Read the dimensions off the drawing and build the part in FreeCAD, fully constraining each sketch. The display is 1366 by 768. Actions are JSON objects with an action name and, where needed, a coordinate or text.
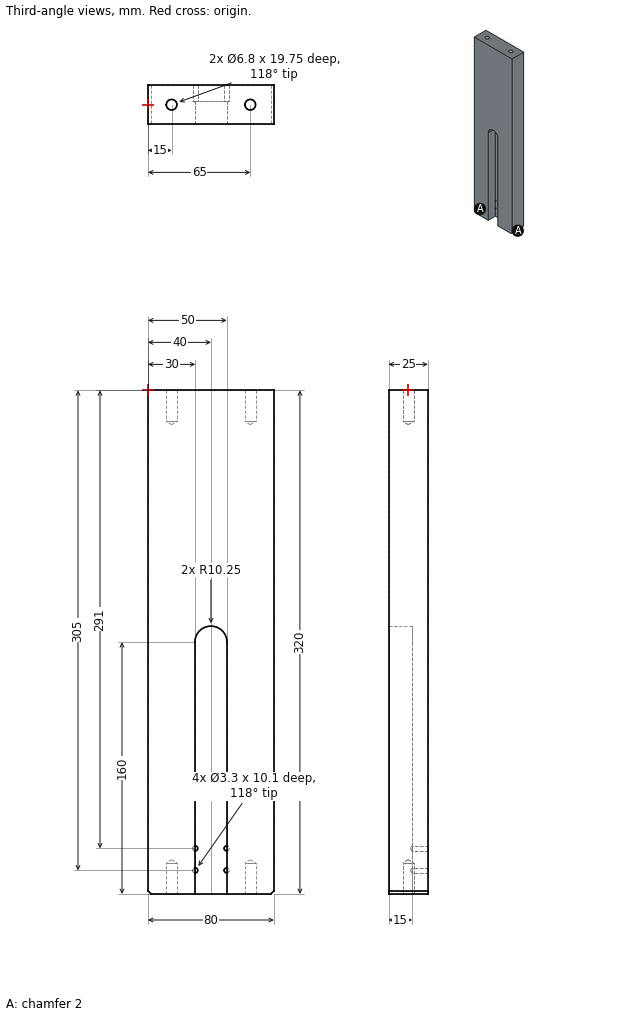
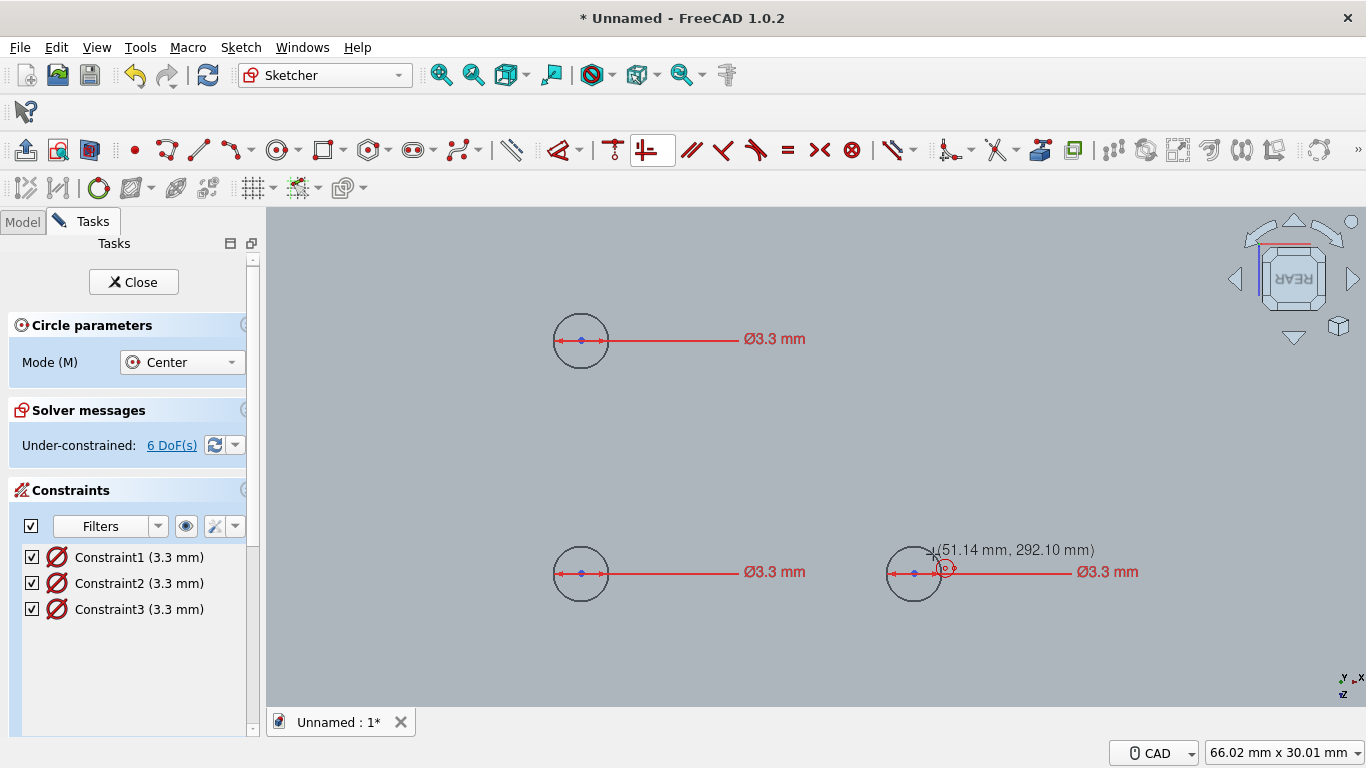
{"action": "left_click", "coordinate": [914, 340]}
{"action": "mouse_move", "coordinate": [933, 321]}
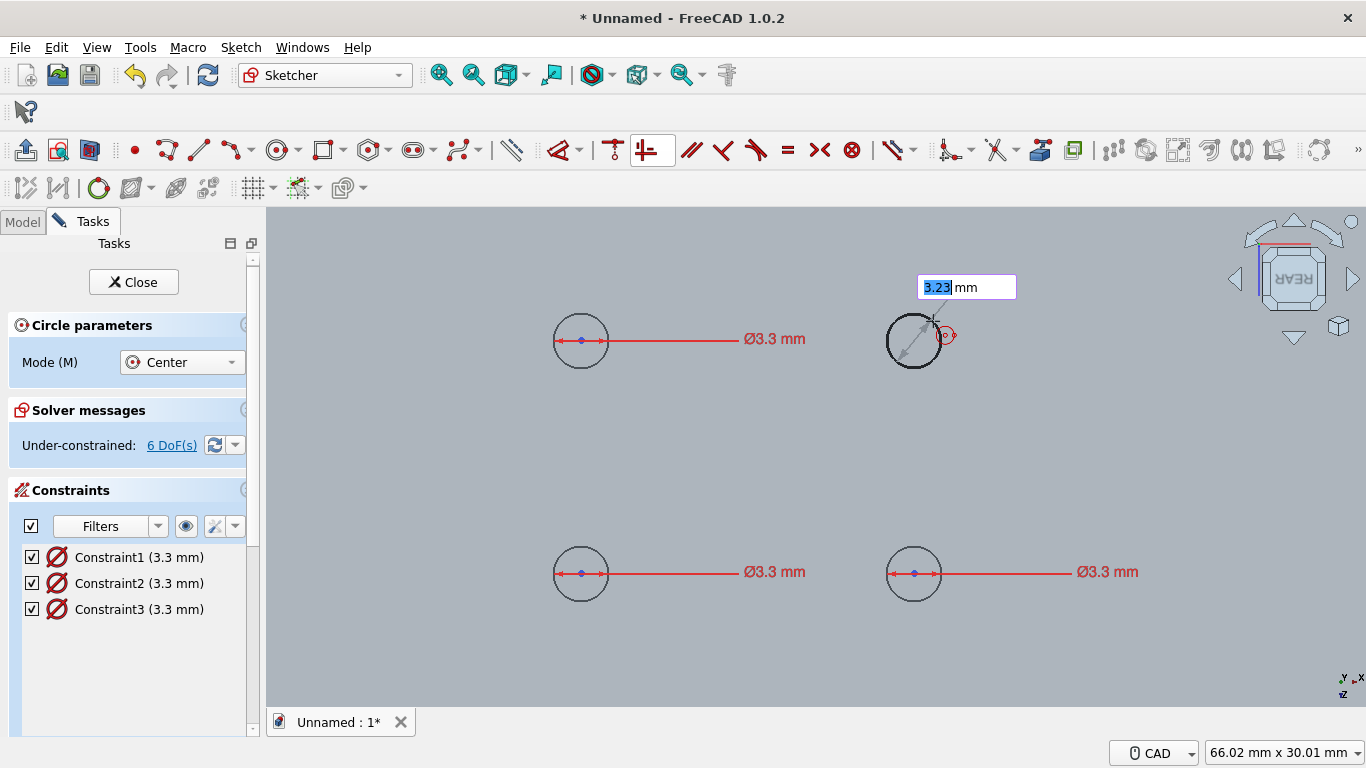
{"action": "type", "text": "3.3"}
{"action": "key", "text": "Return"}
{"action": "key", "text": "Escape"}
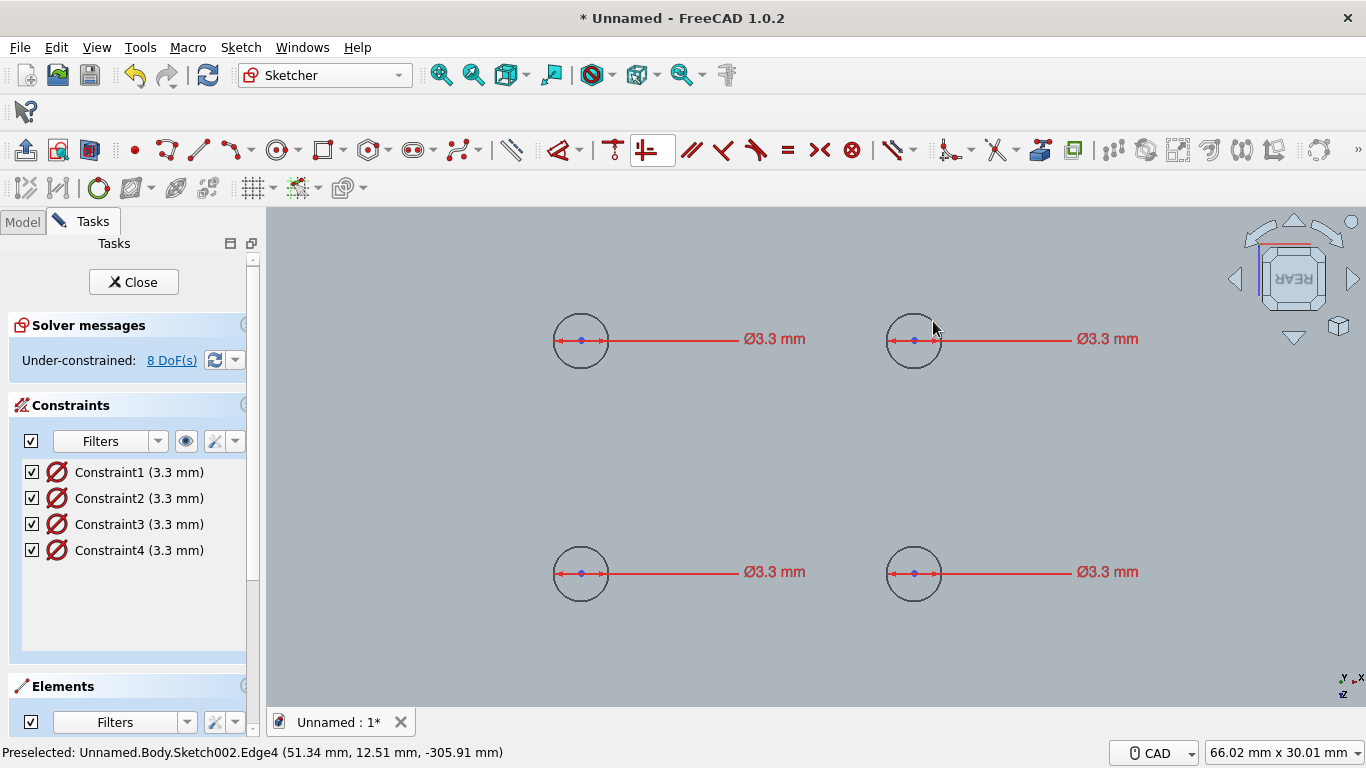
{"action": "left_click", "coordinate": [581, 341]}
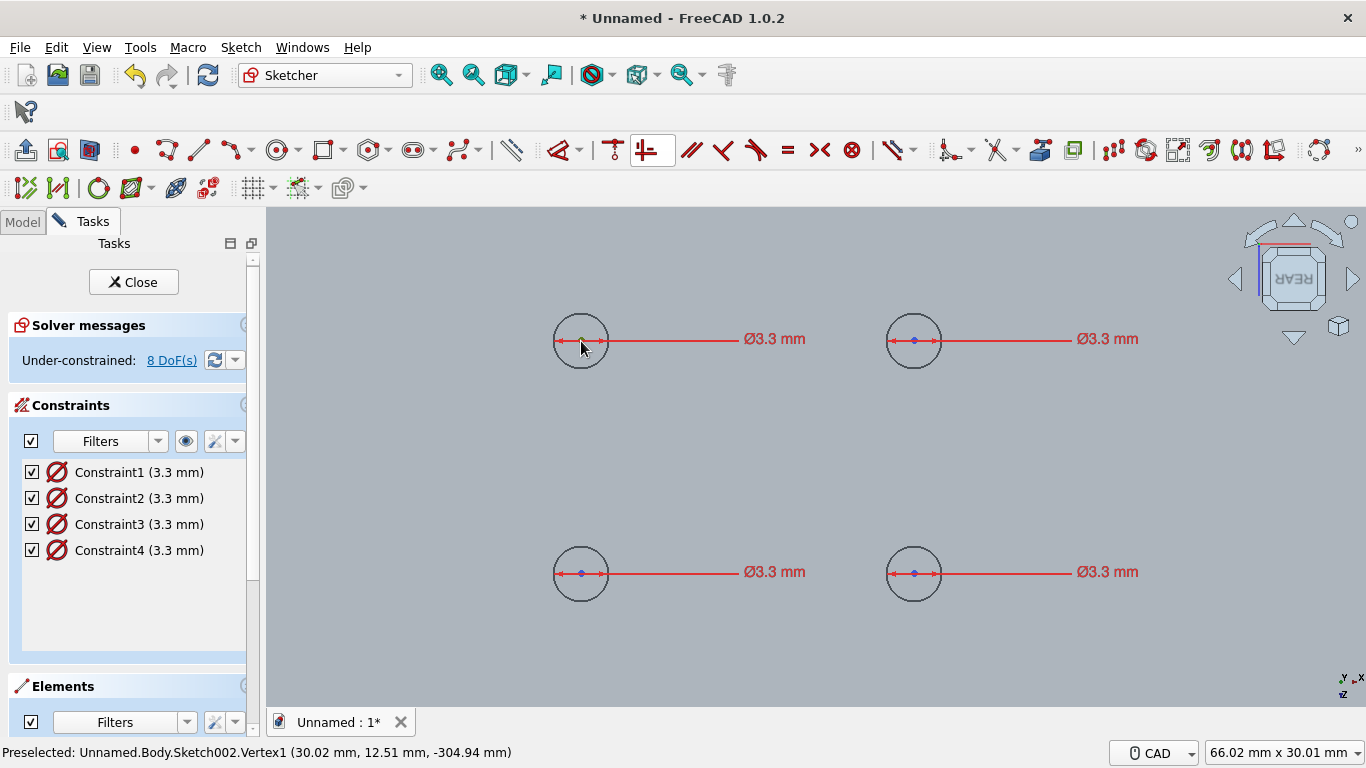
{"action": "left_click", "coordinate": [581, 574]}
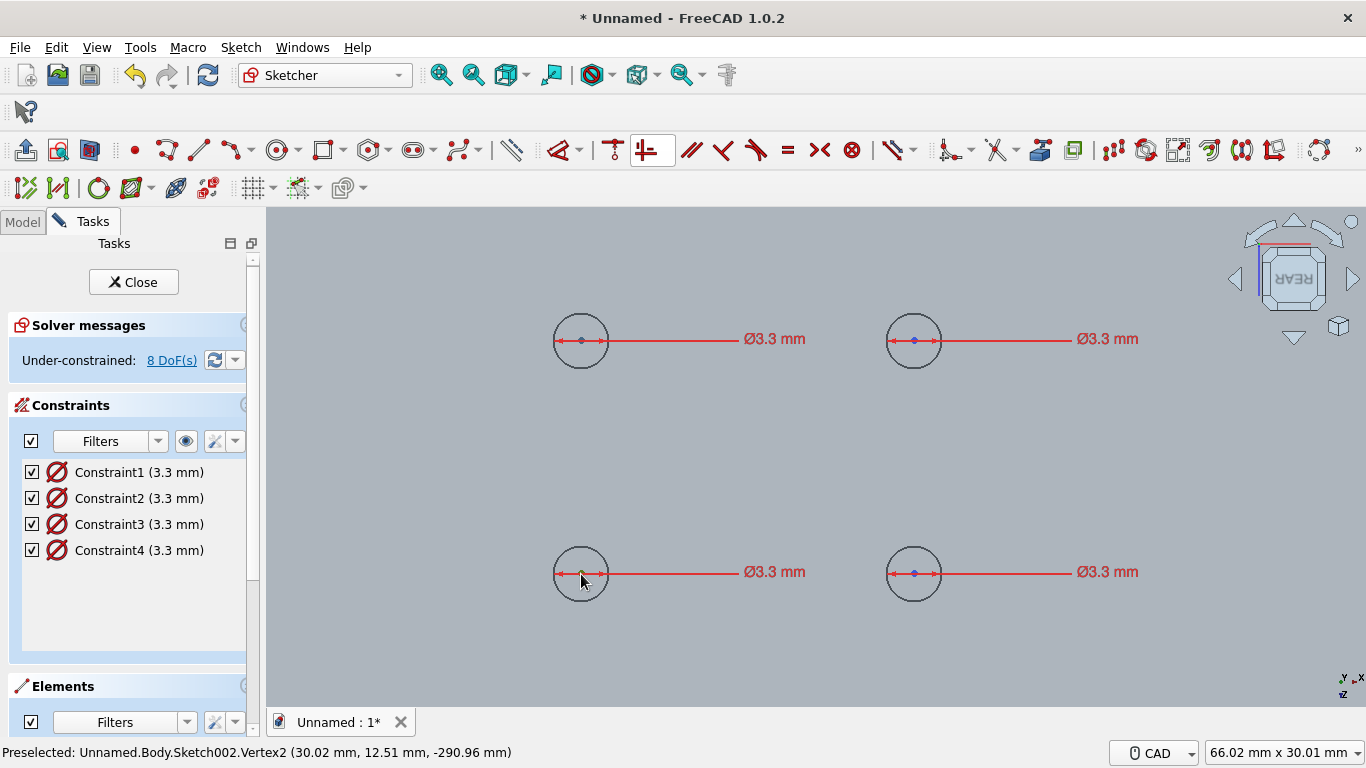
{"action": "left_click", "coordinate": [670, 150]}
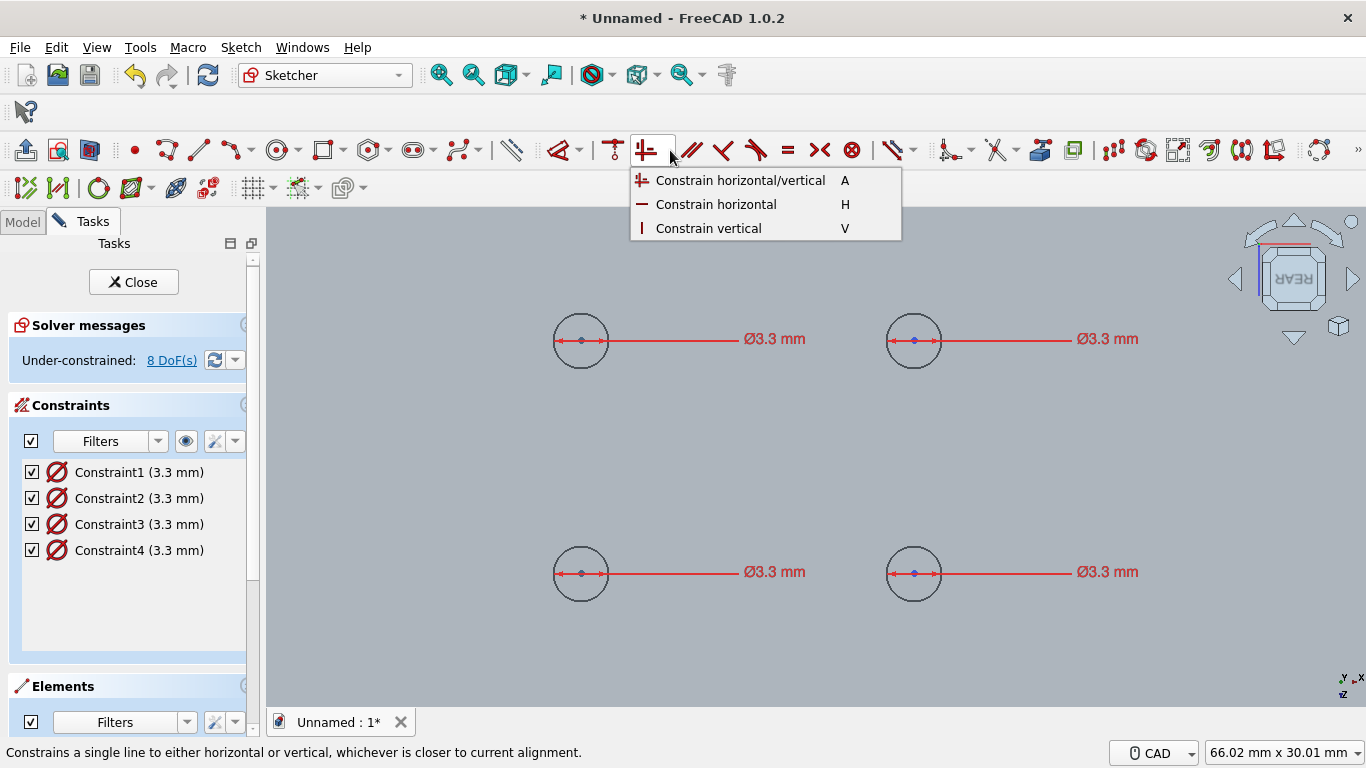
{"action": "left_click", "coordinate": [766, 228]}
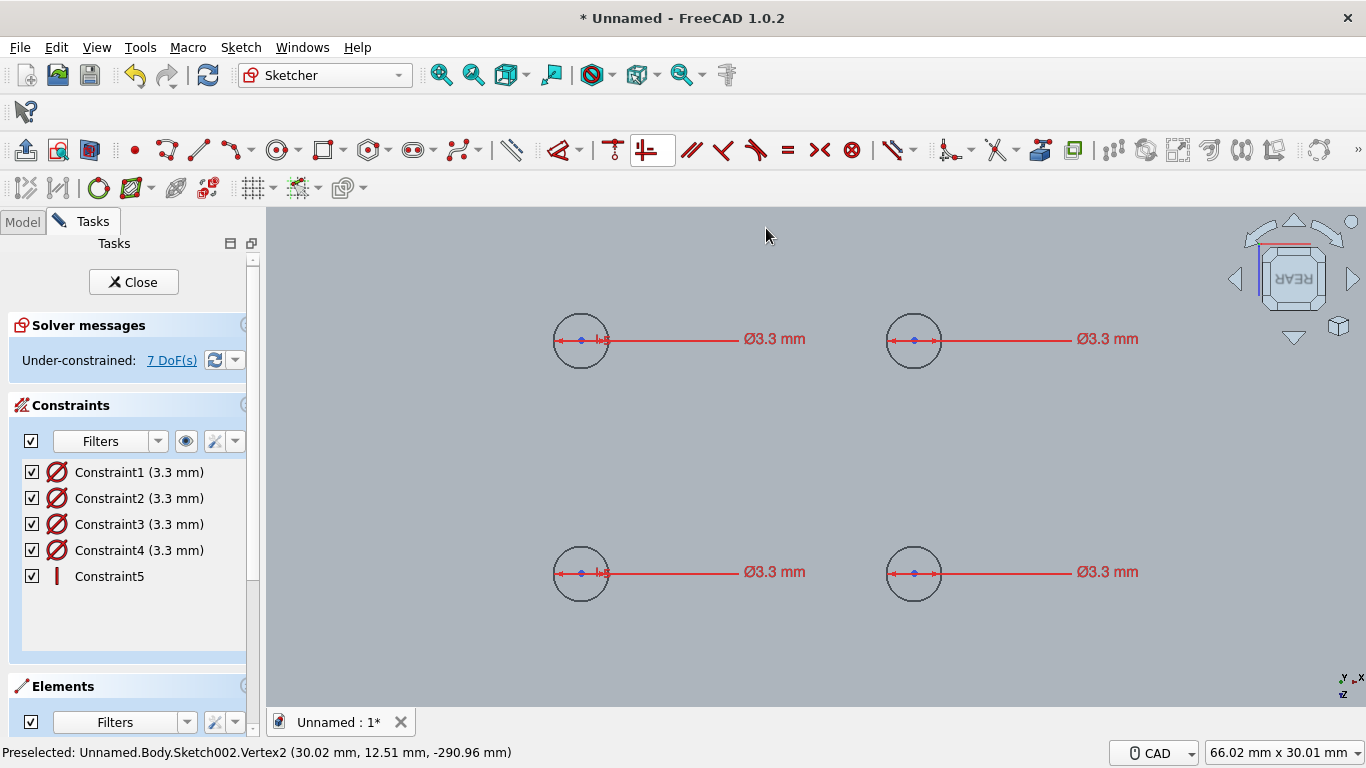
{"action": "left_click", "coordinate": [581, 574]}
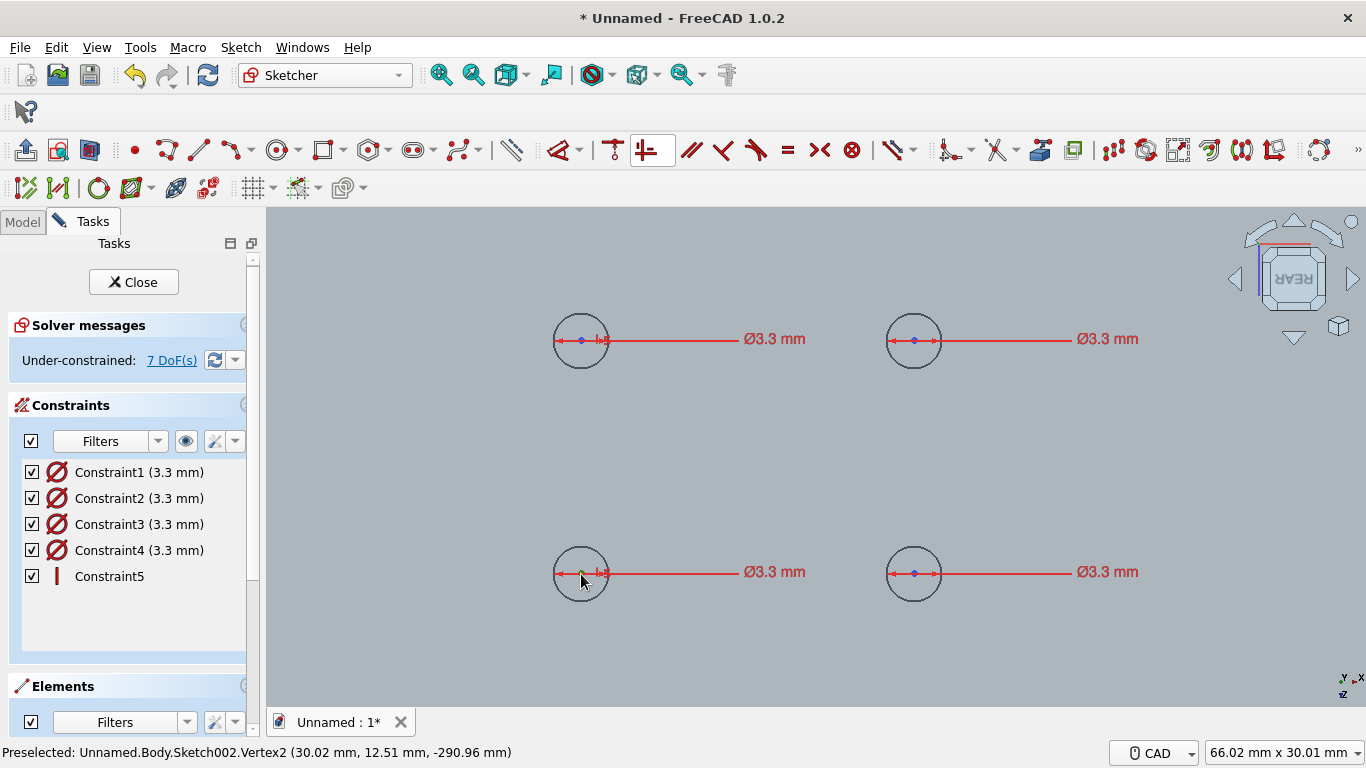
{"action": "left_click", "coordinate": [914, 574]}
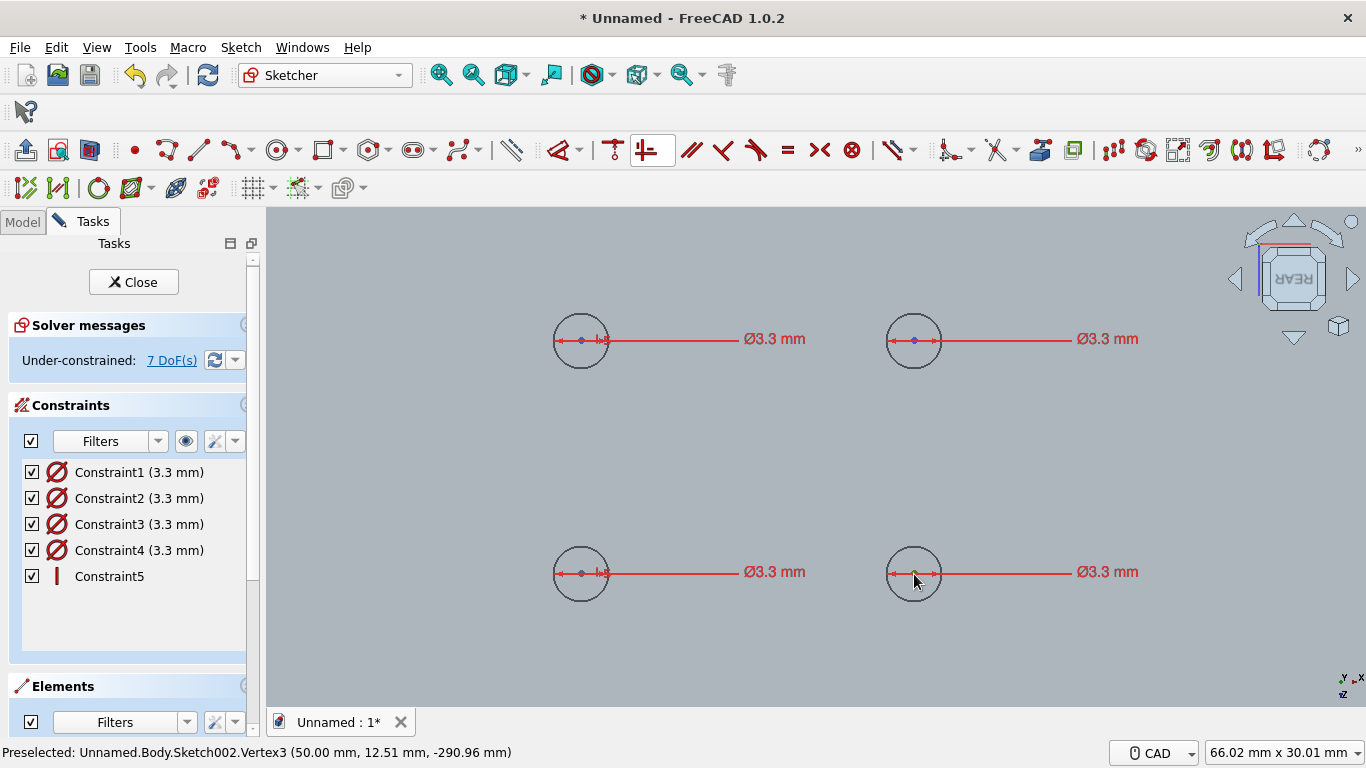
{"action": "key", "text": "h"}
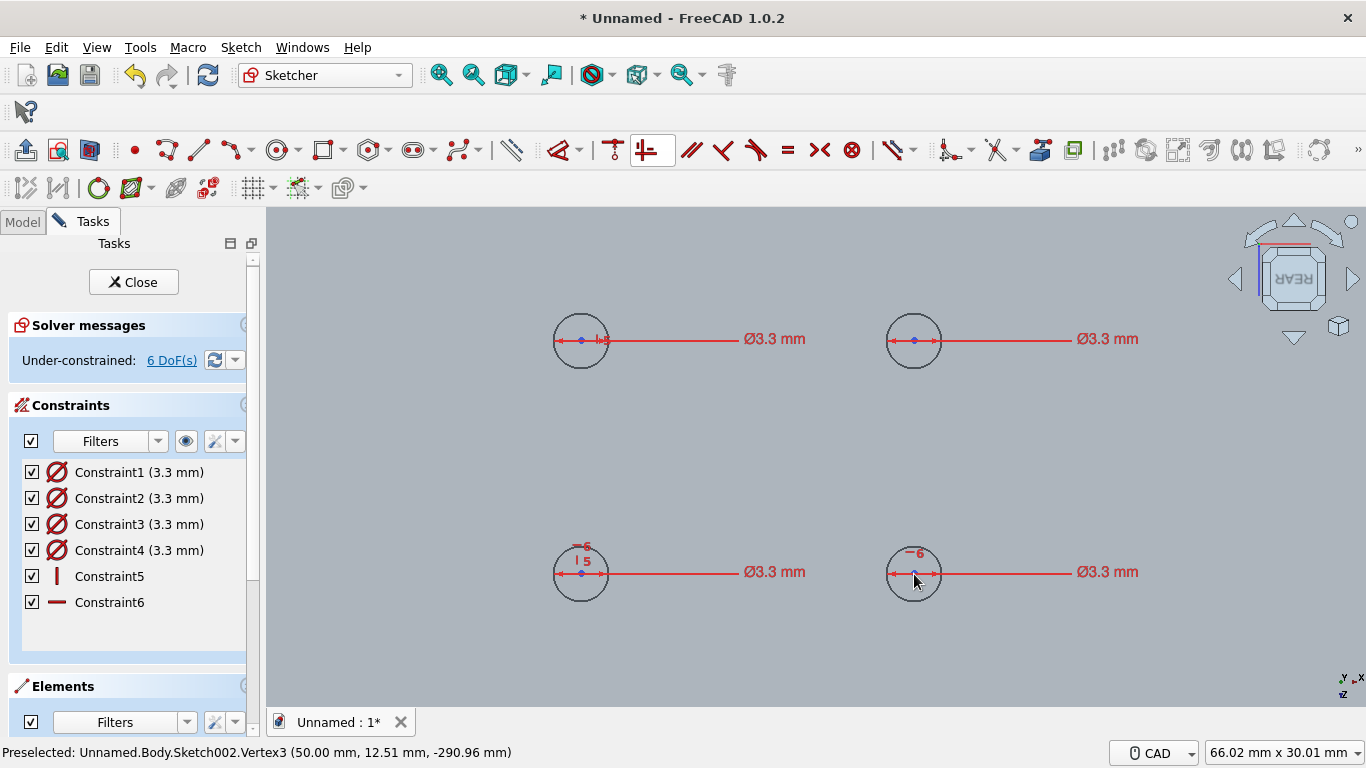
{"action": "left_click", "coordinate": [914, 574]}